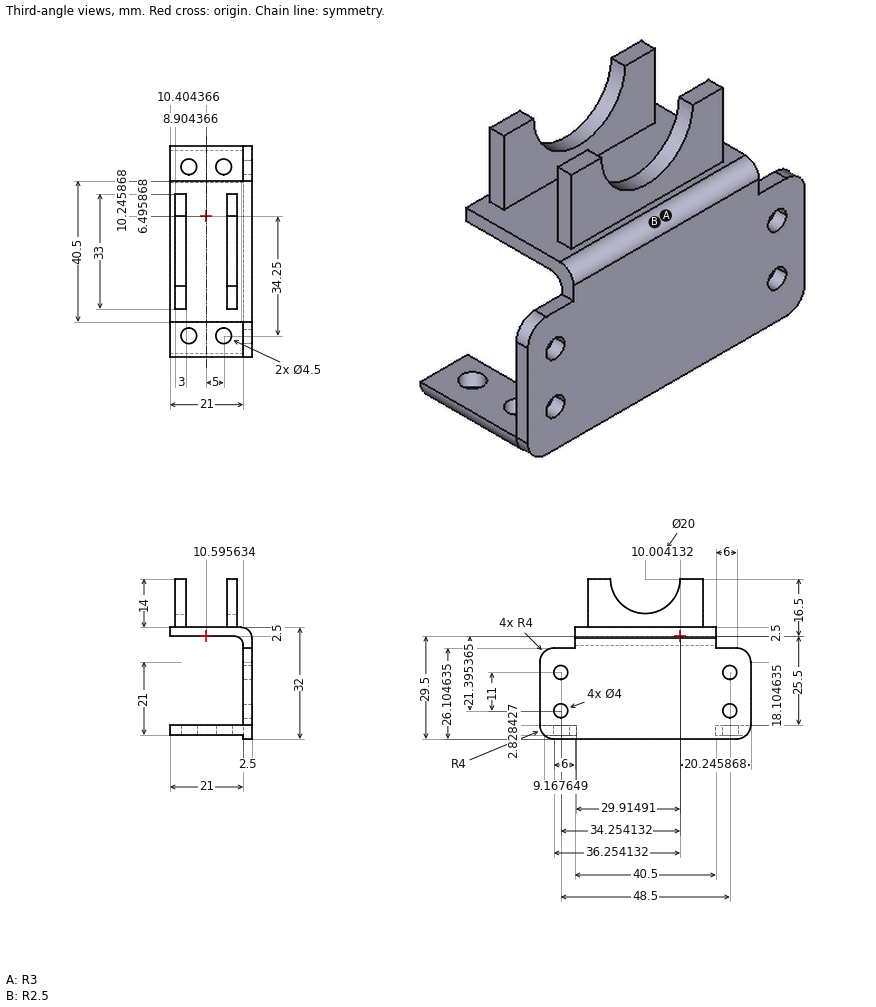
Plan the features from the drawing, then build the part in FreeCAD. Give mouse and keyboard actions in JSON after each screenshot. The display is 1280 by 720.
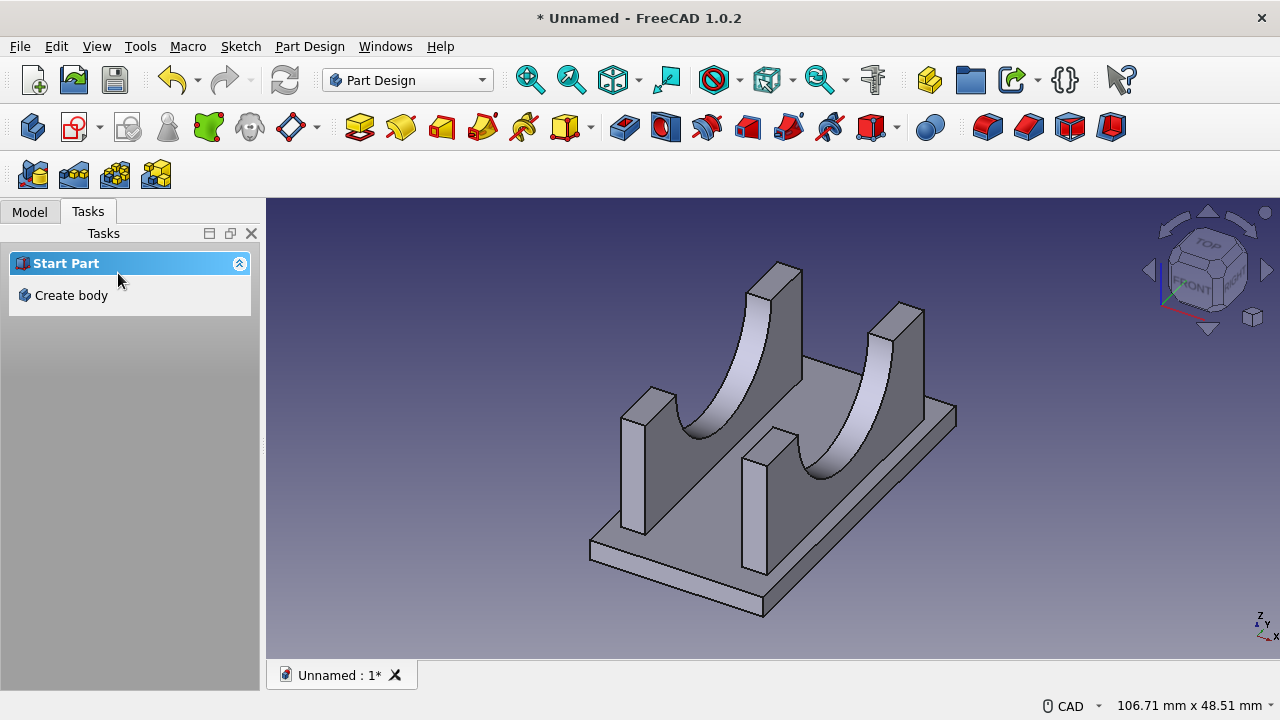
{"action": "left_click", "coordinate": [30, 212]}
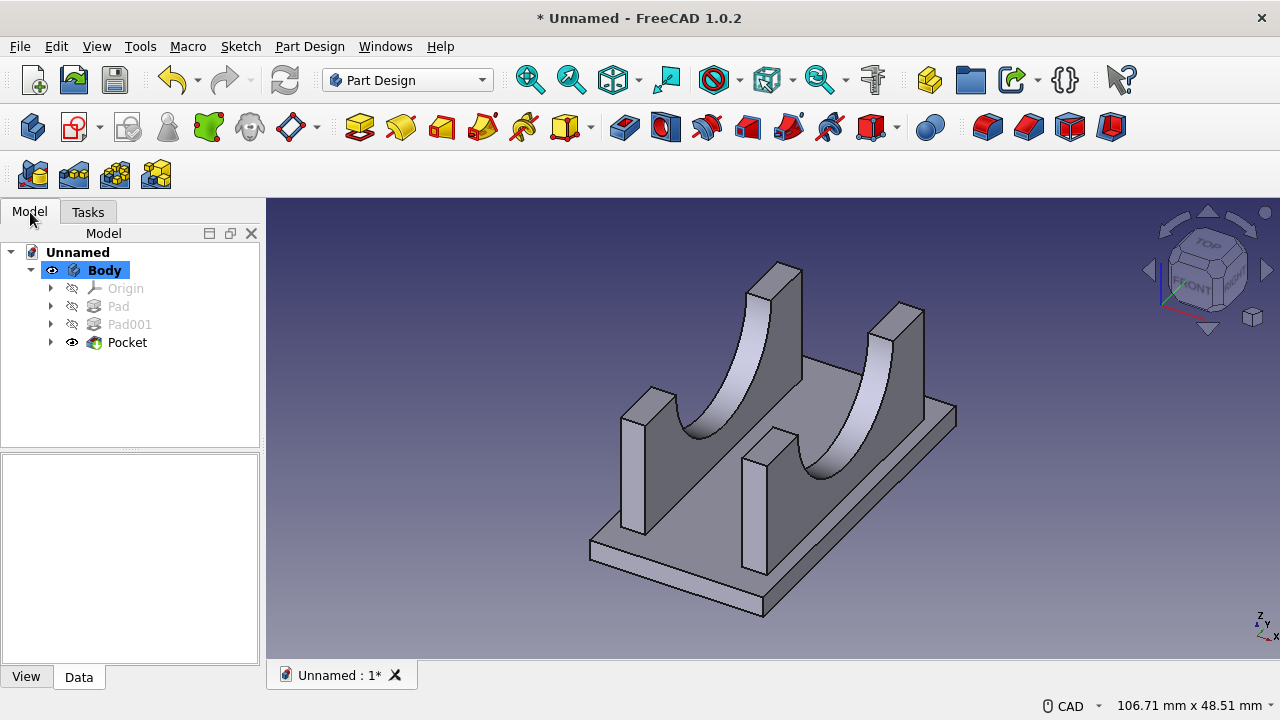
{"action": "left_click", "coordinate": [51, 288]}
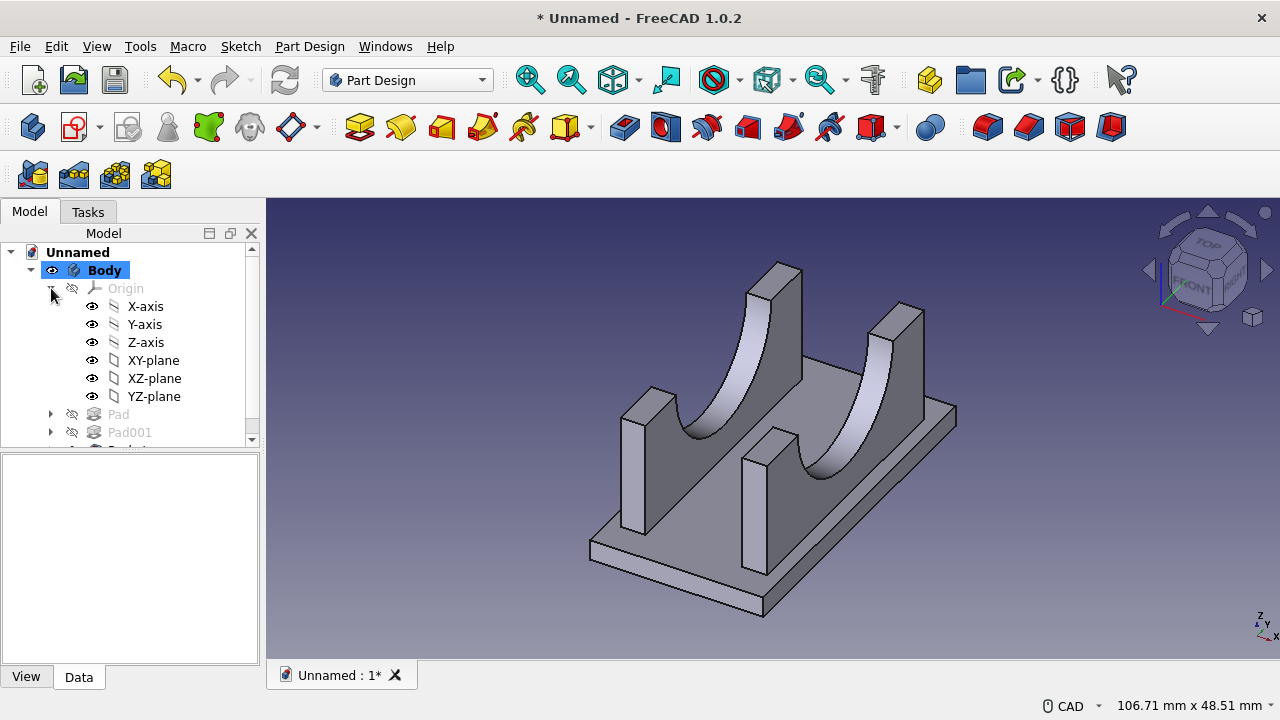
{"action": "left_click", "coordinate": [137, 378]}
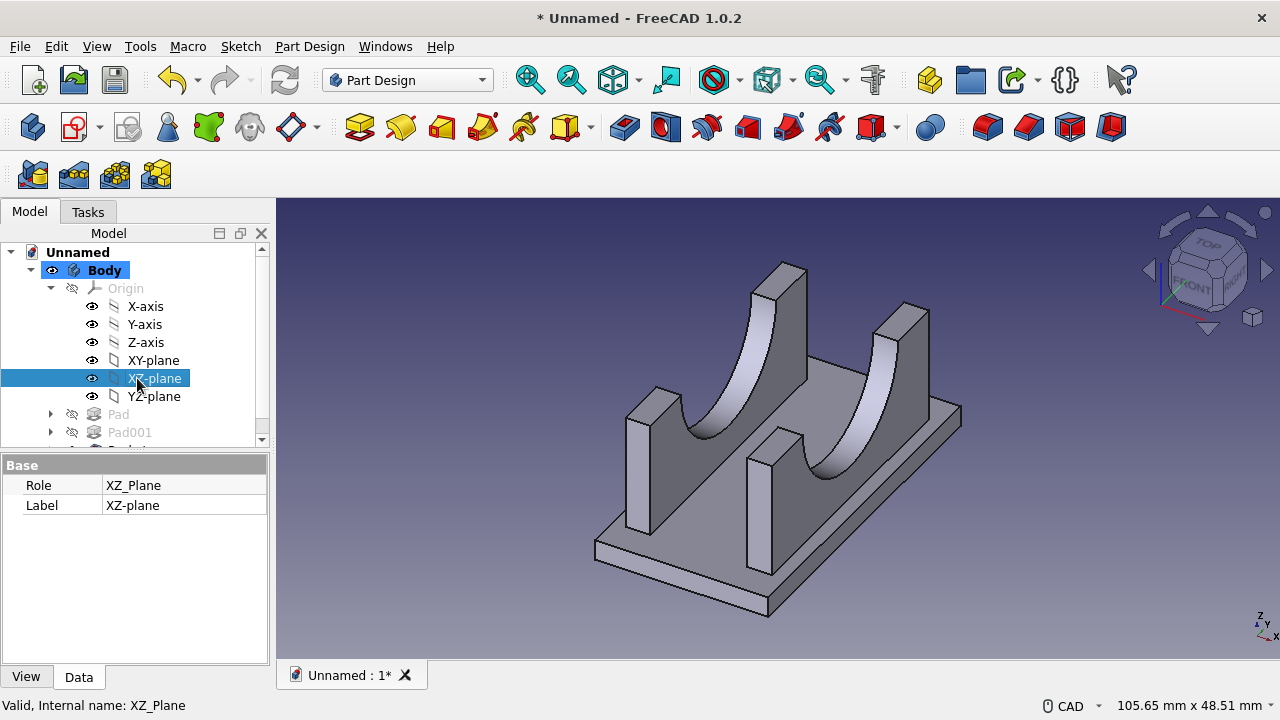
{"action": "left_click", "coordinate": [290, 128]}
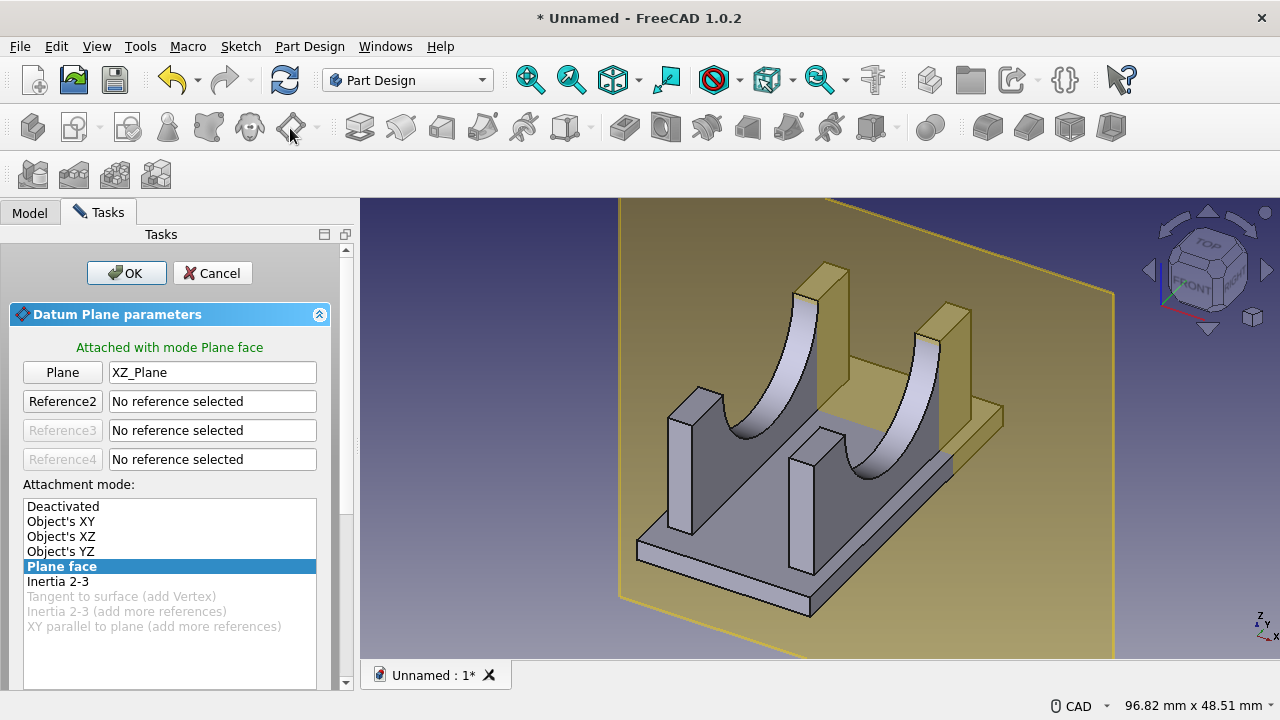
{"action": "scroll", "coordinate": [346, 467], "scroll_direction": "down", "scroll_amount": 4}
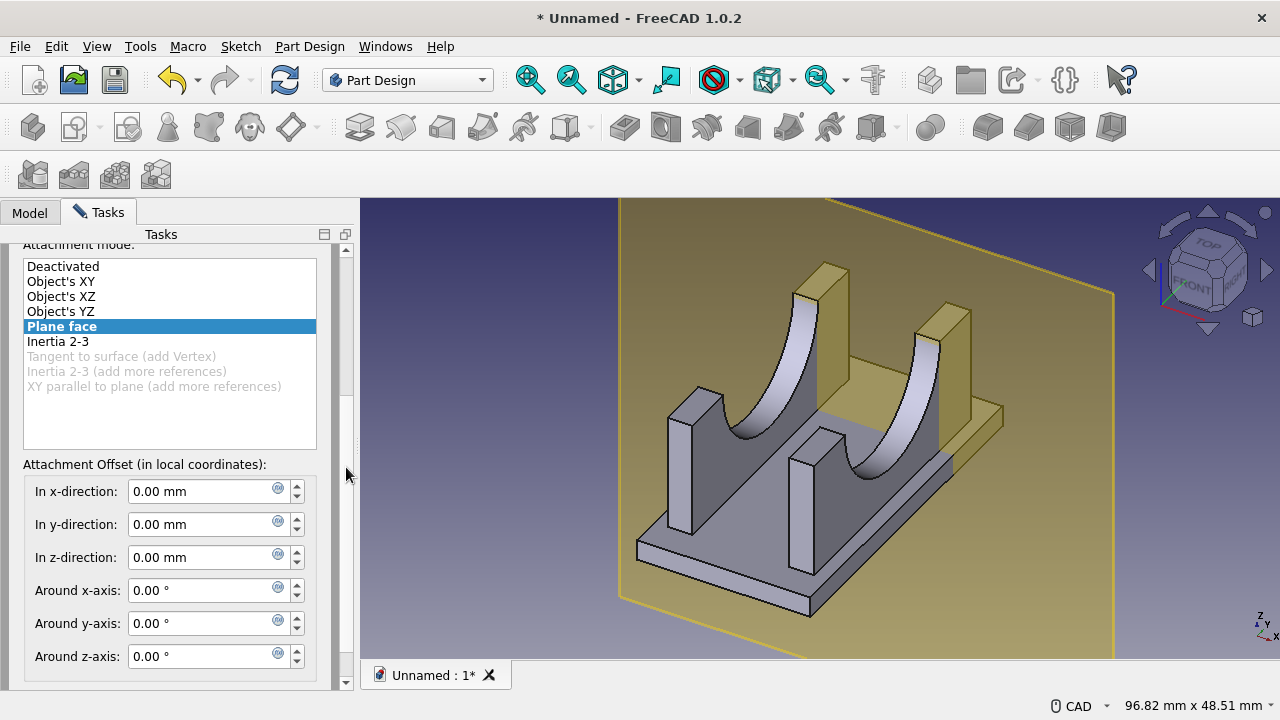
{"action": "triple_click", "coordinate": [210, 558]}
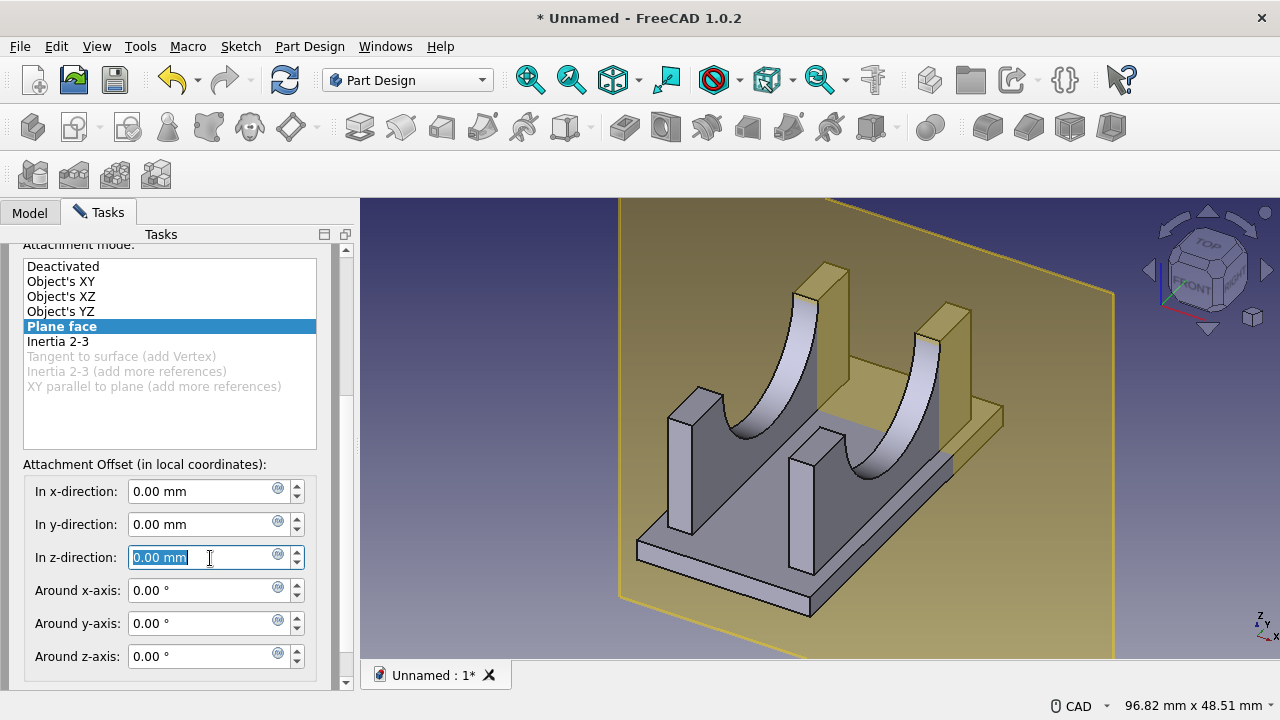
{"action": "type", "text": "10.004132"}
{"action": "key", "text": "Tab"}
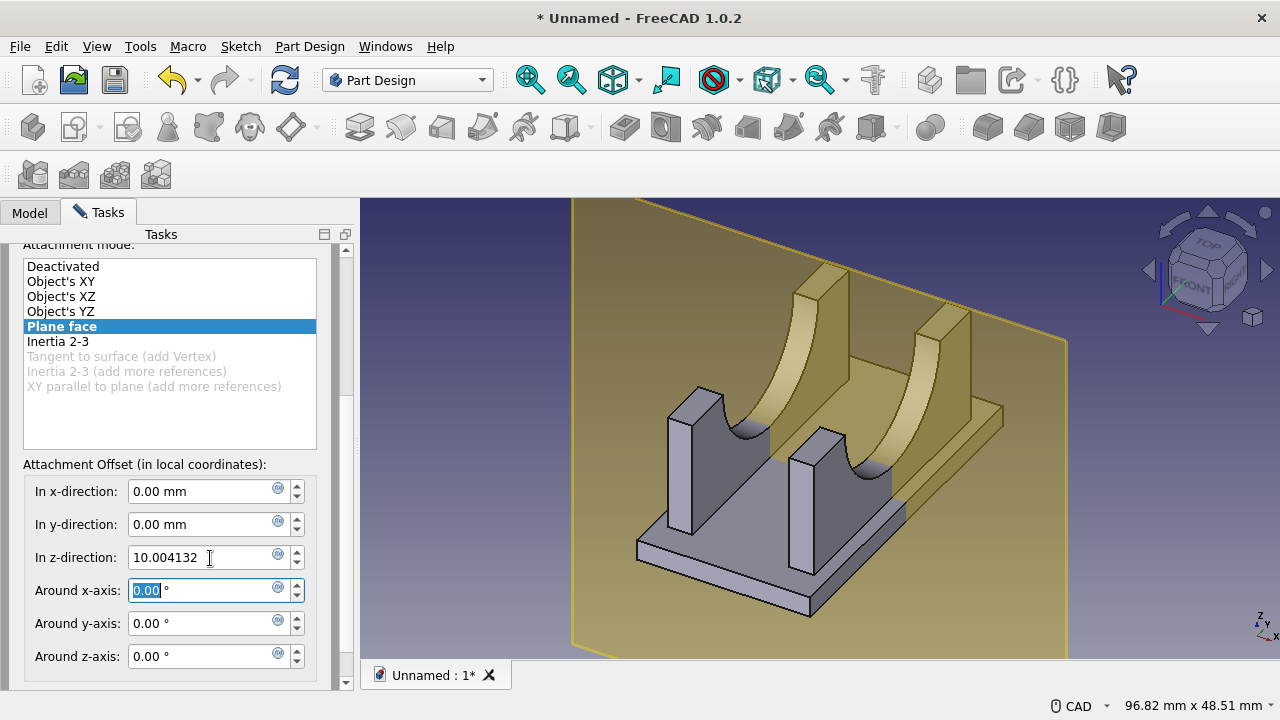
{"action": "scroll", "coordinate": [346, 467], "scroll_direction": "up", "scroll_amount": 5}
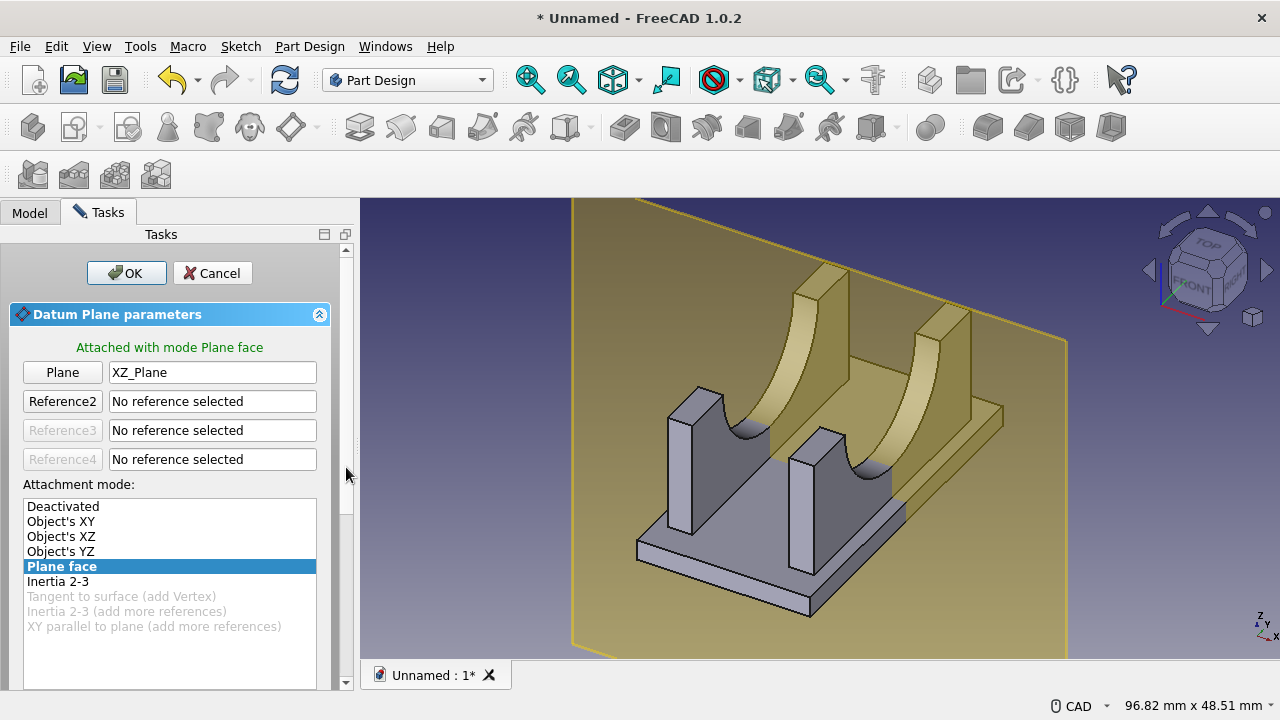
{"action": "left_click", "coordinate": [127, 273]}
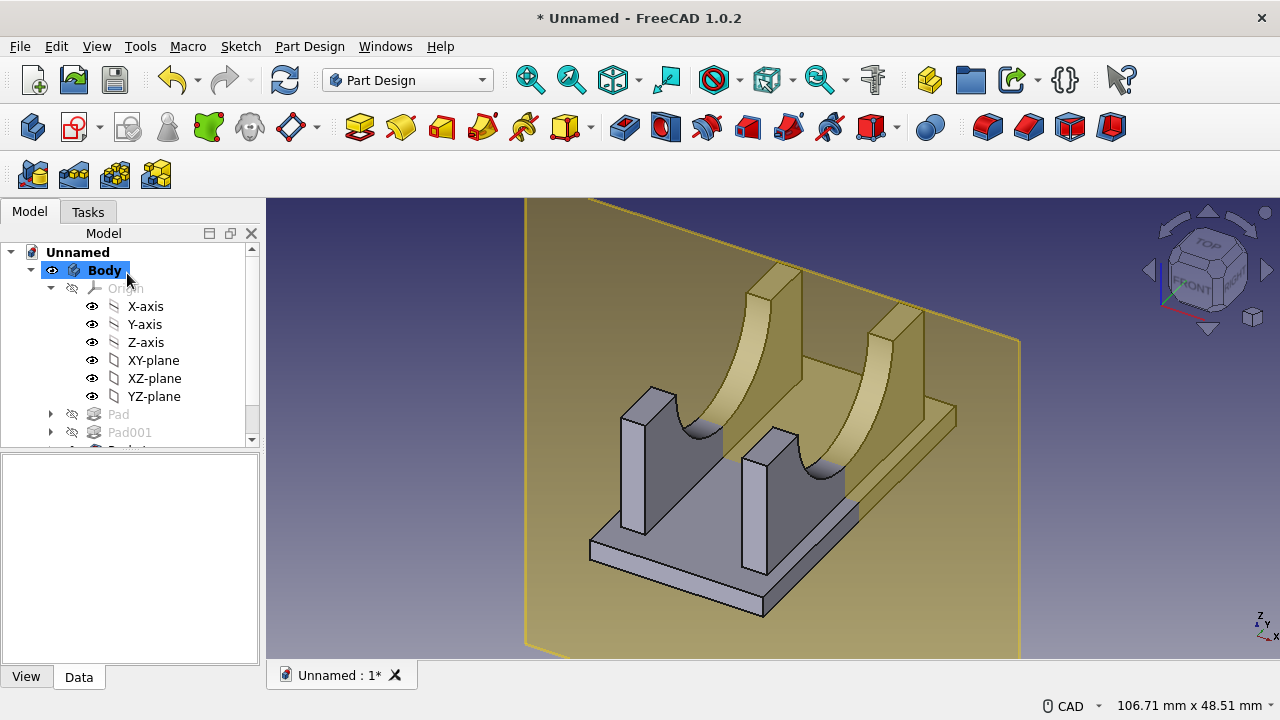
{"action": "scroll", "coordinate": [101, 338], "scroll_direction": "down", "scroll_amount": 3}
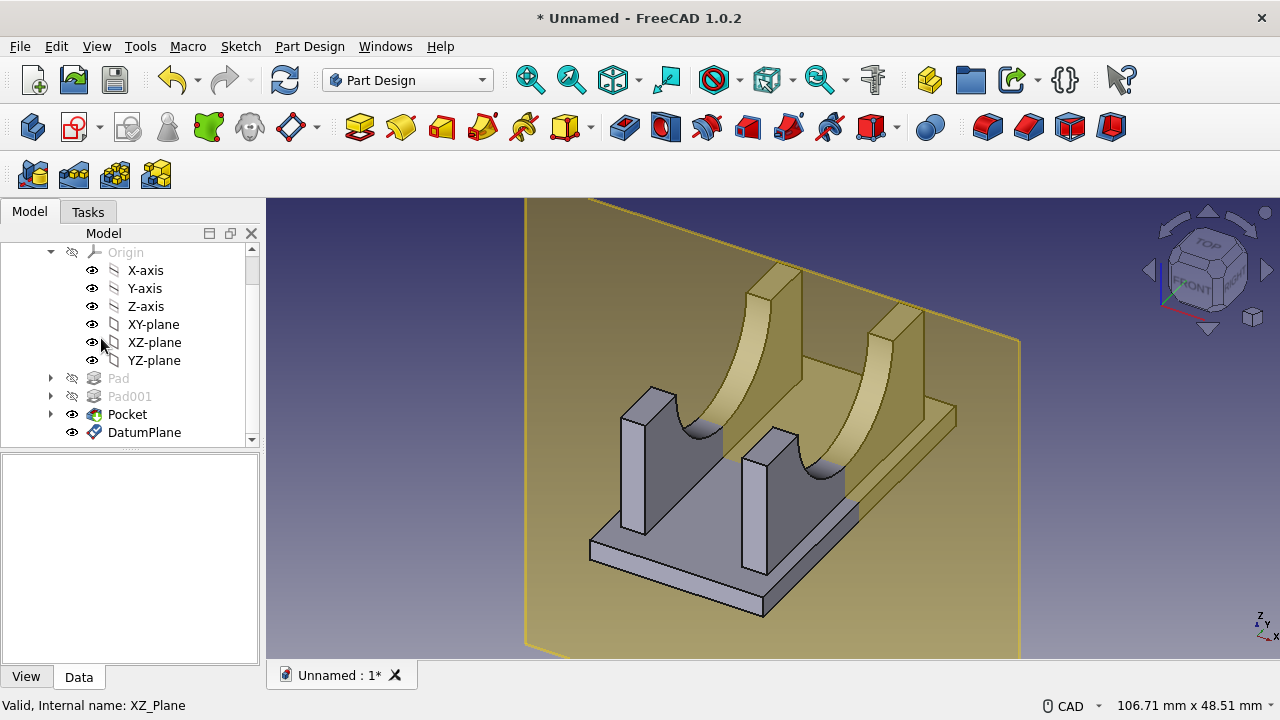
{"action": "left_click", "coordinate": [117, 432]}